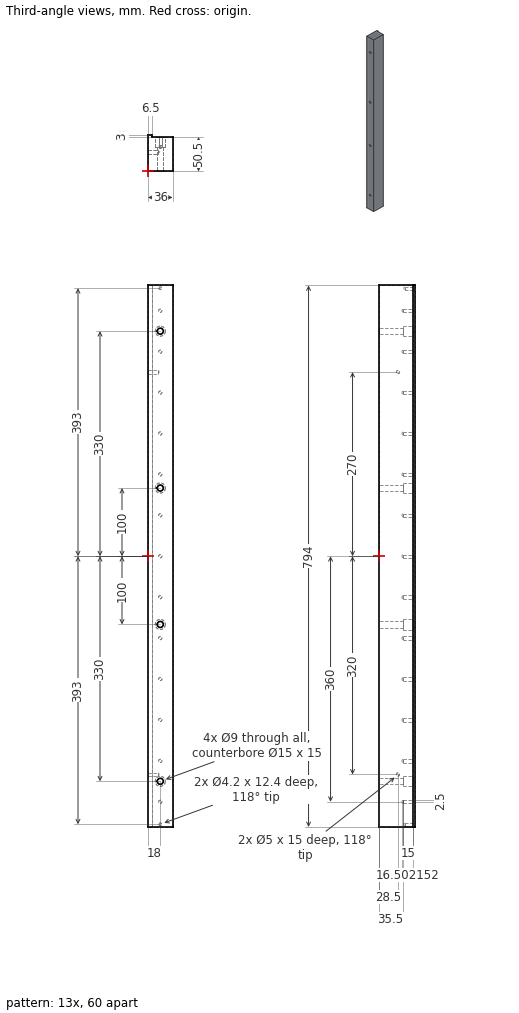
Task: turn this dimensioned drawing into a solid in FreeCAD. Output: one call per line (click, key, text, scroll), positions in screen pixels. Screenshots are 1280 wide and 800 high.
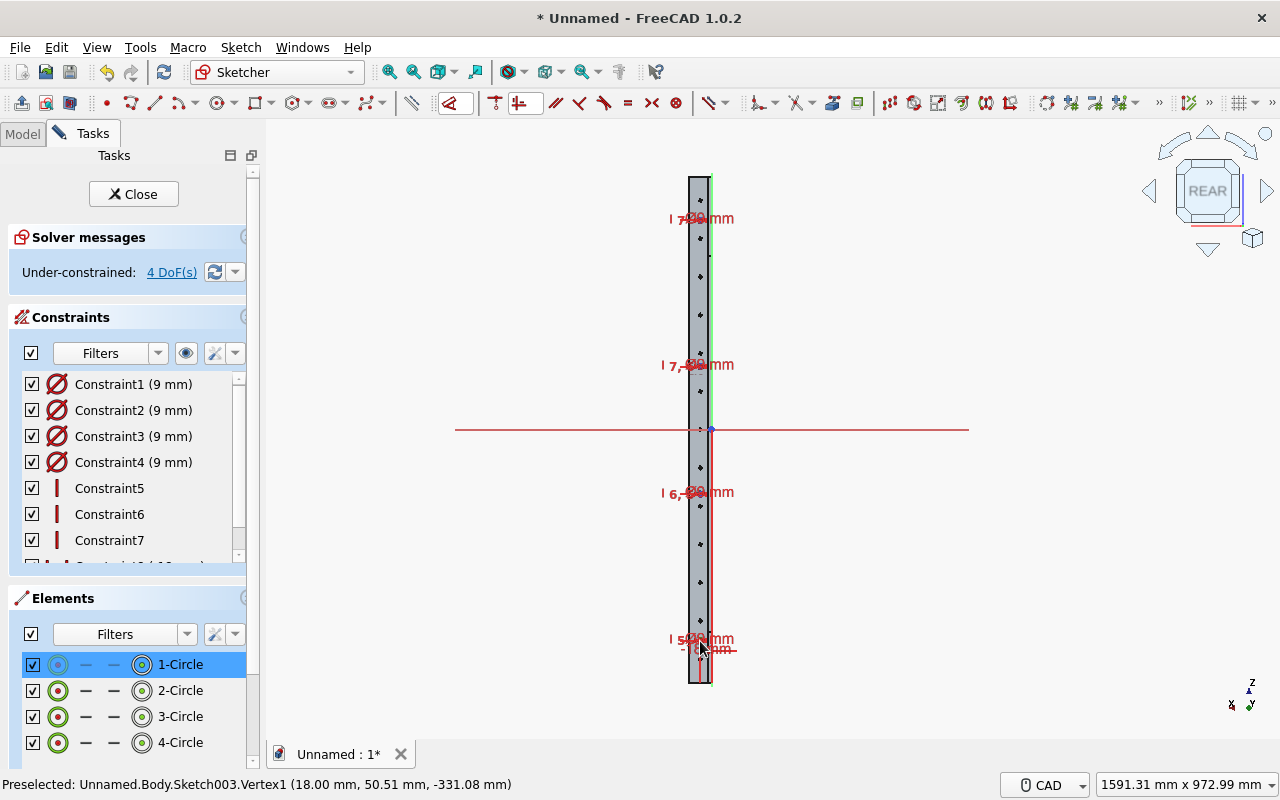
key(i)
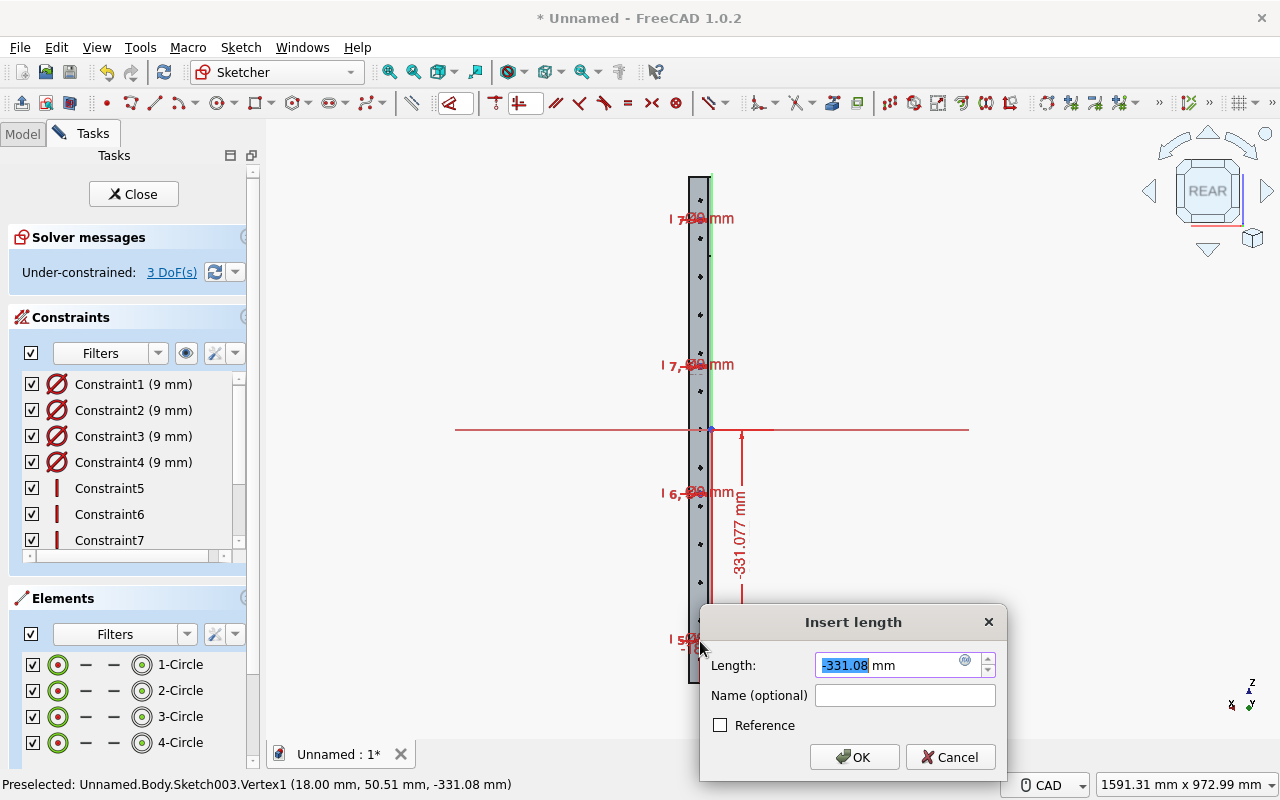
text(-330)
key(Return)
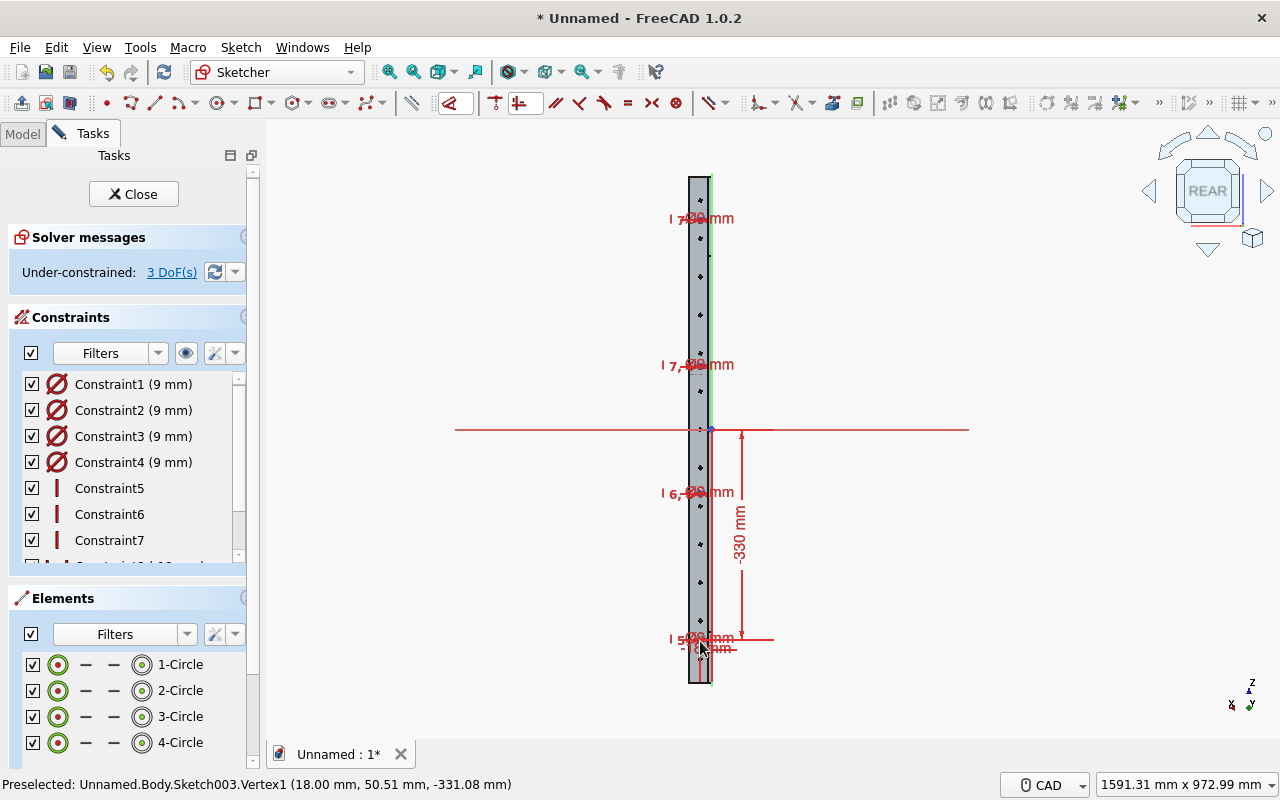
click(700, 494)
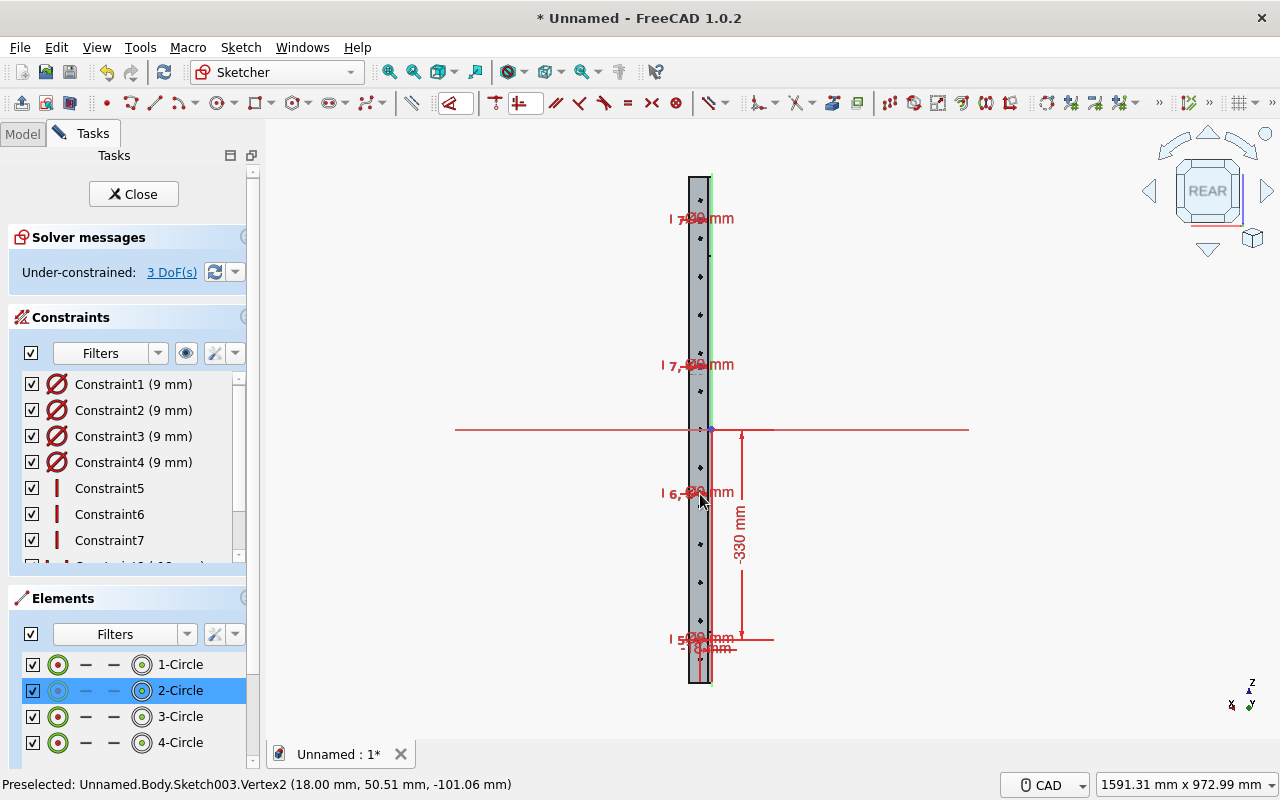
click(468, 104)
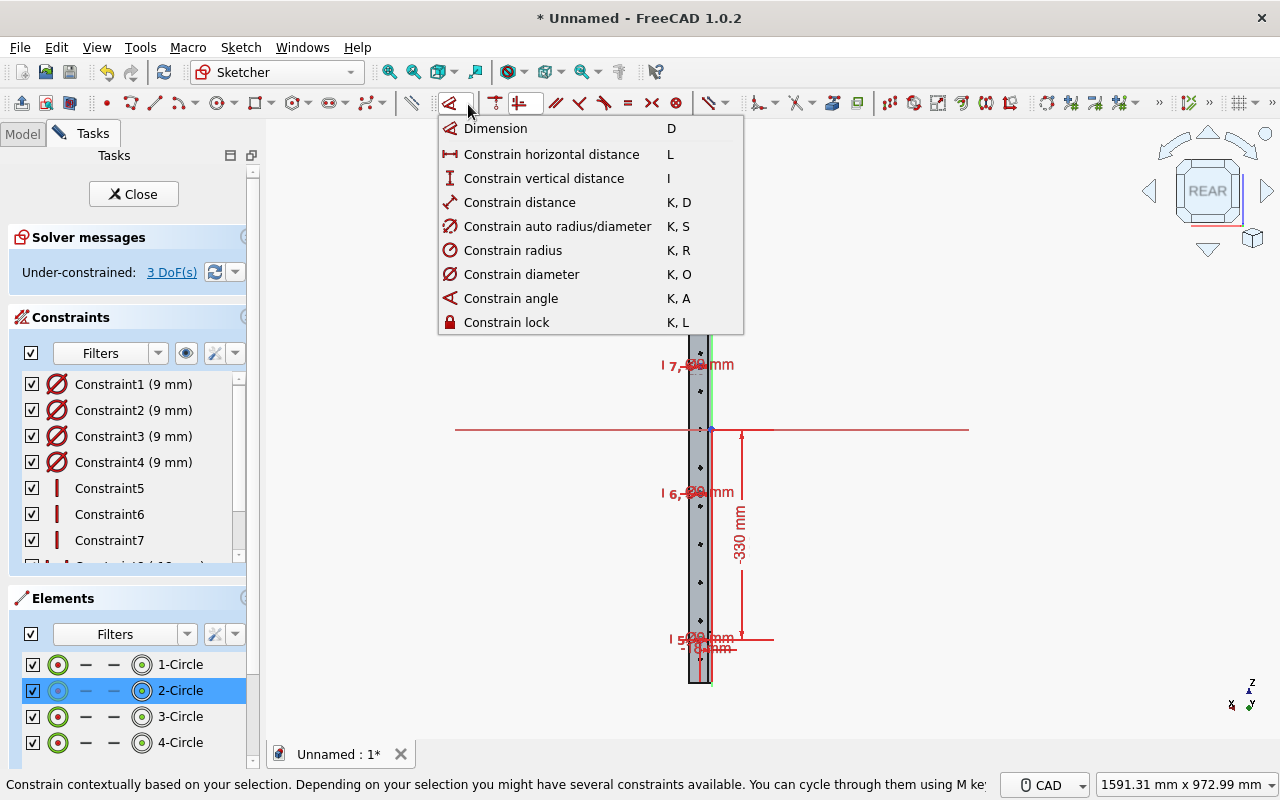
click(591, 178)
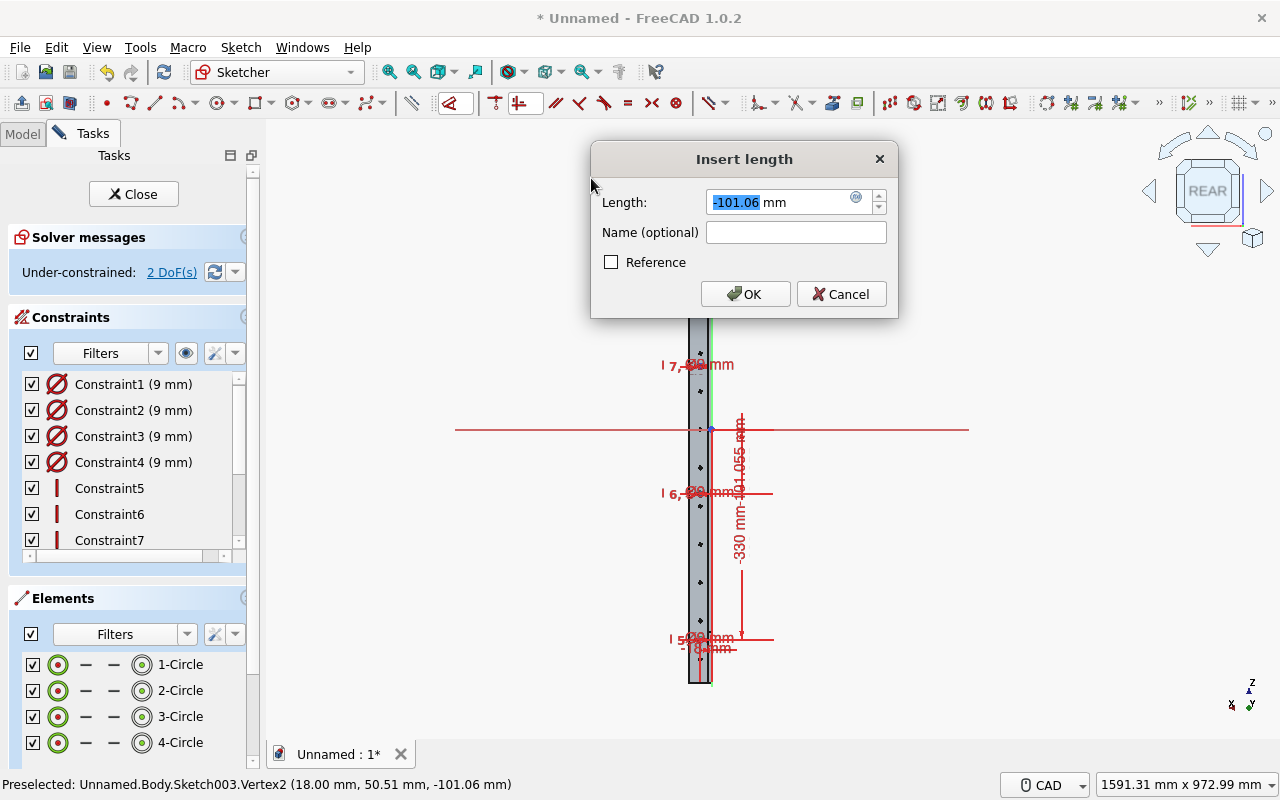
text(-100)
key(Return)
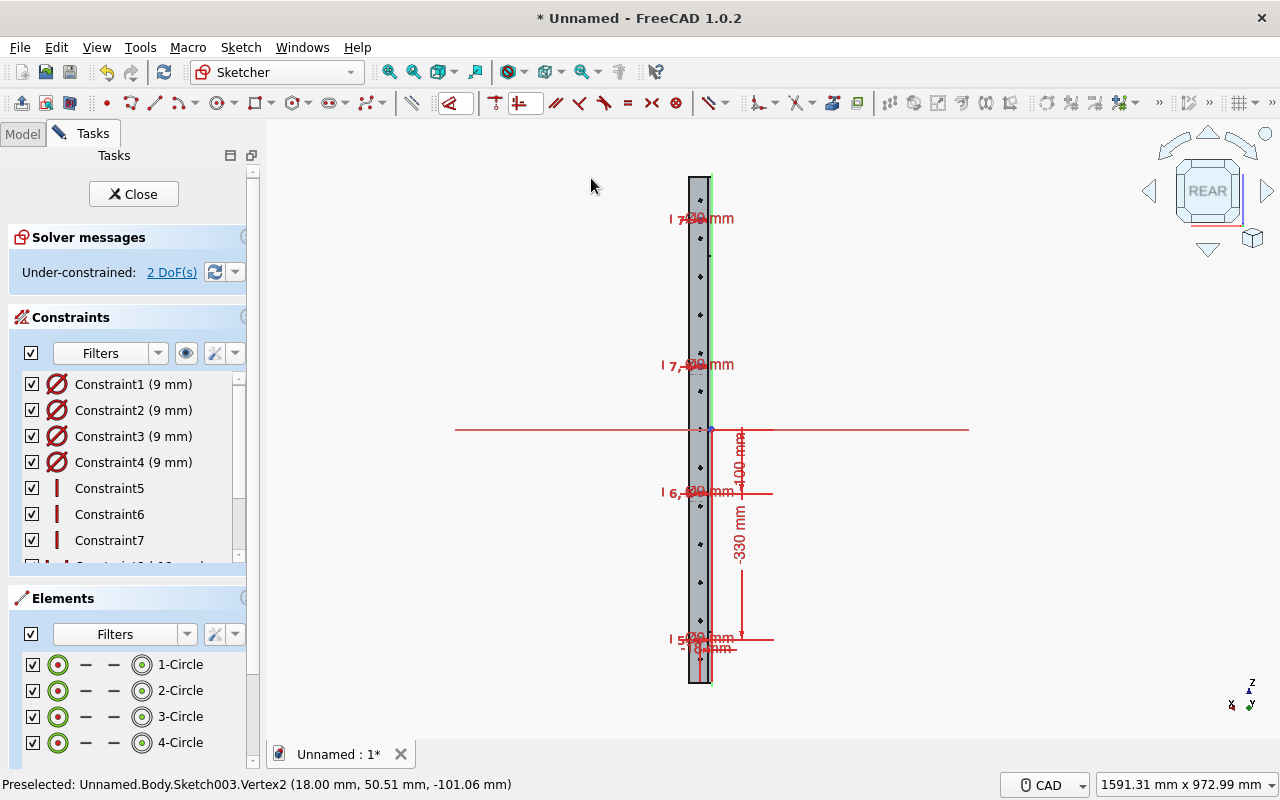
click(700, 367)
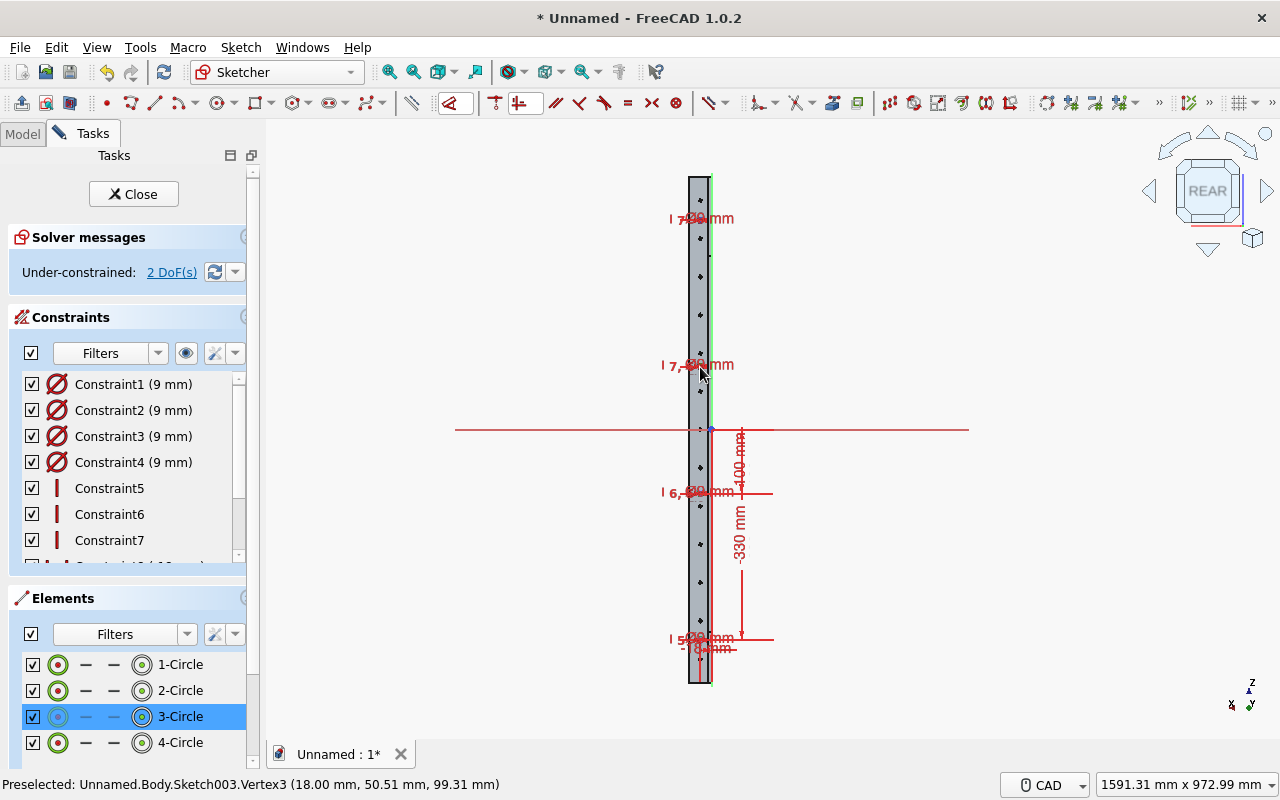
click(468, 104)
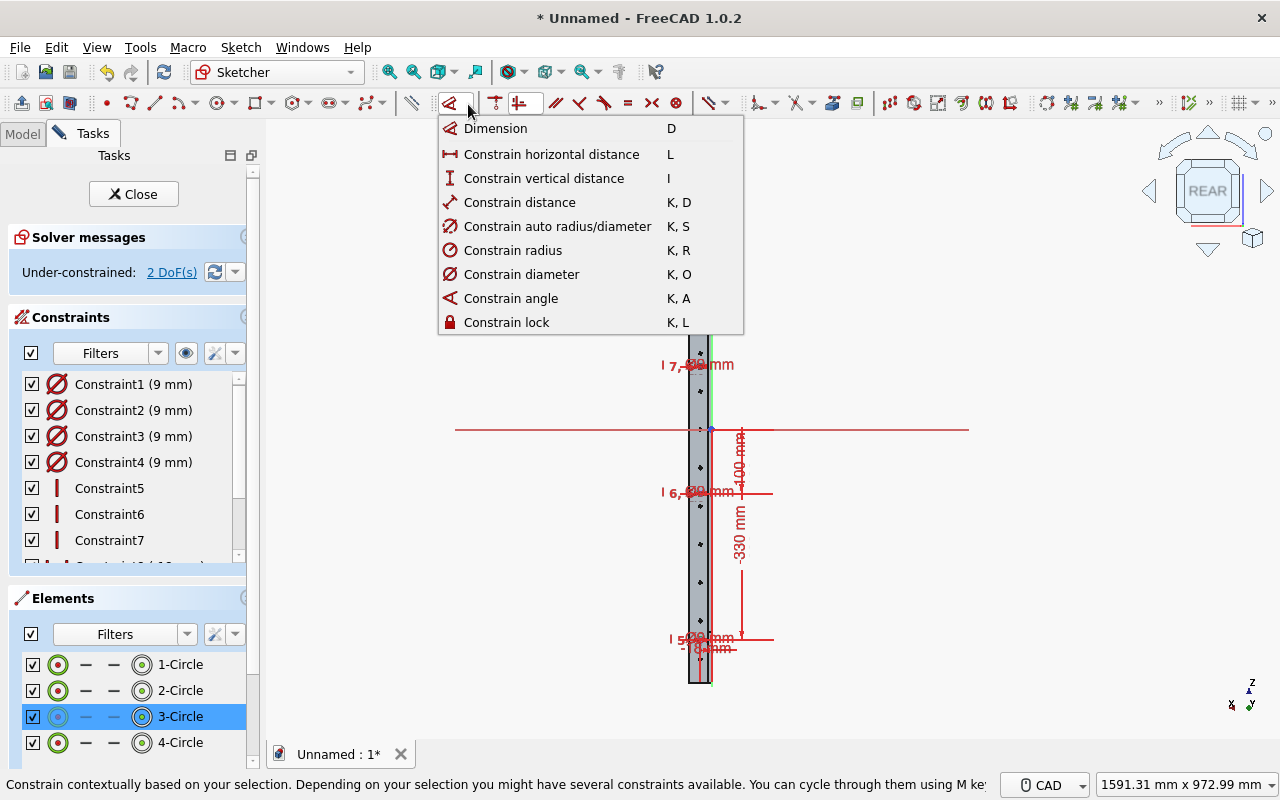
click(591, 178)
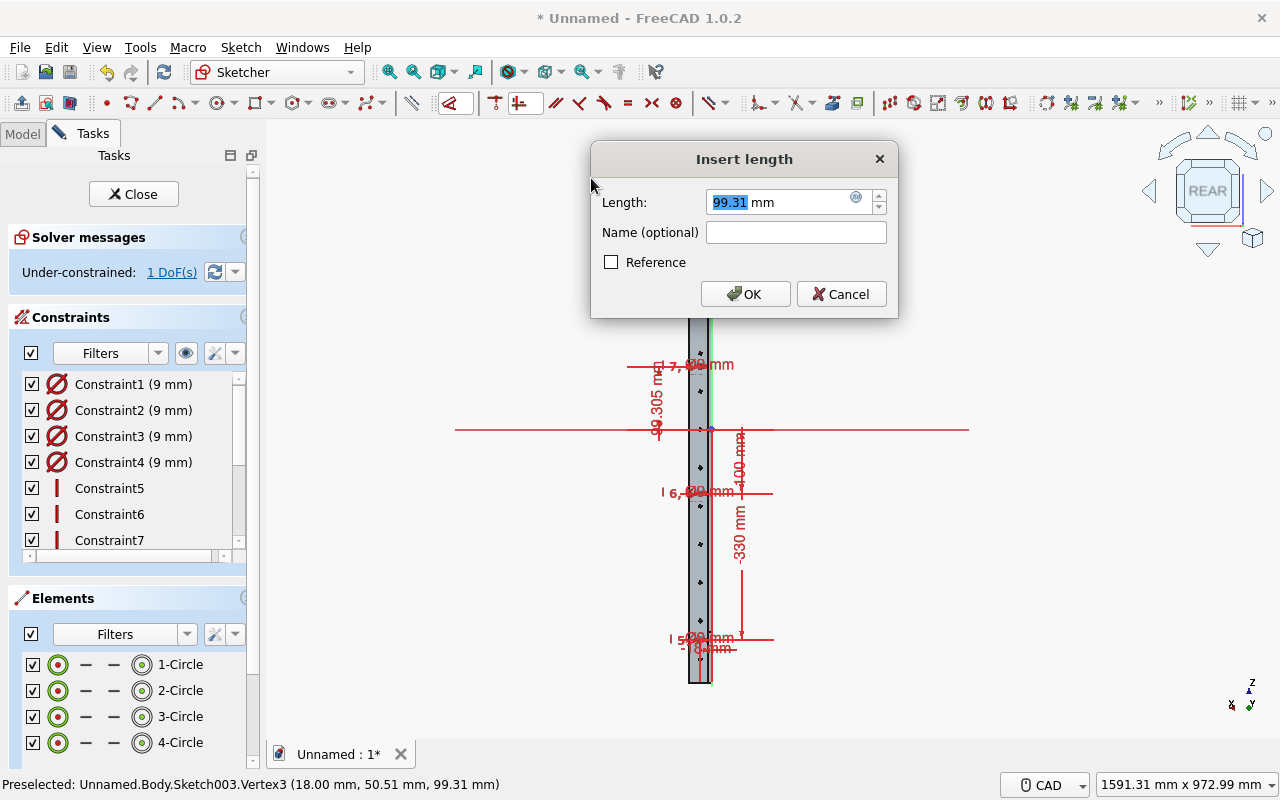
text(100)
key(Return)